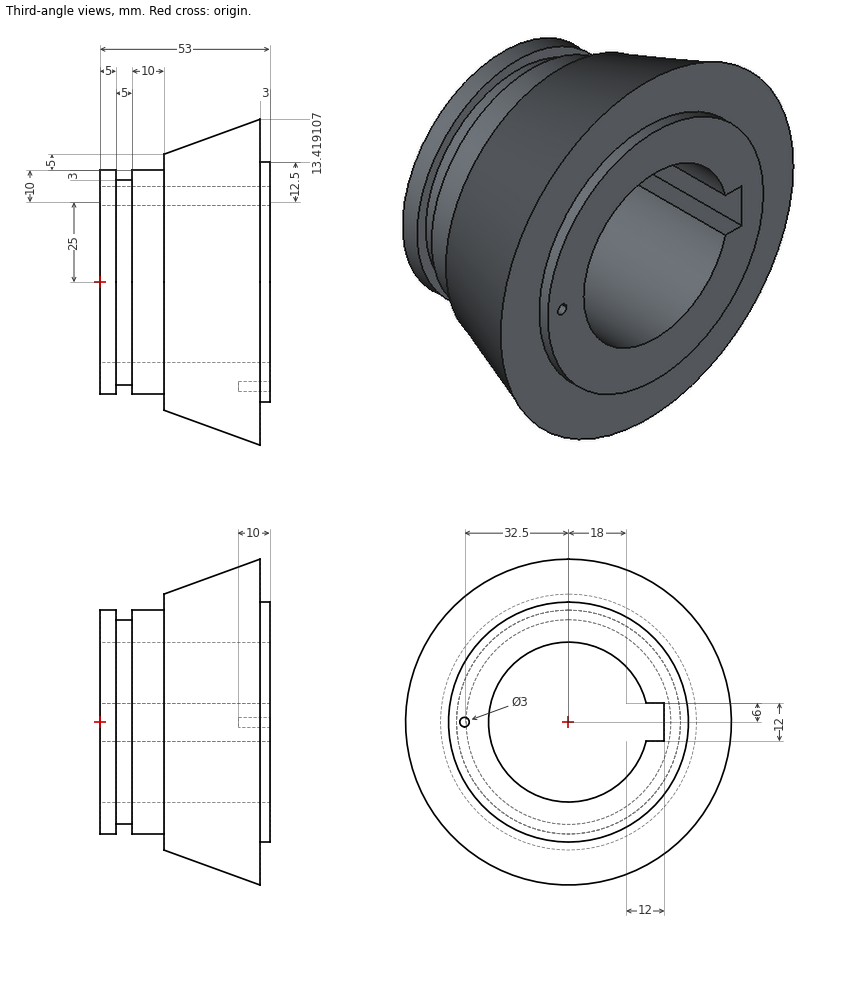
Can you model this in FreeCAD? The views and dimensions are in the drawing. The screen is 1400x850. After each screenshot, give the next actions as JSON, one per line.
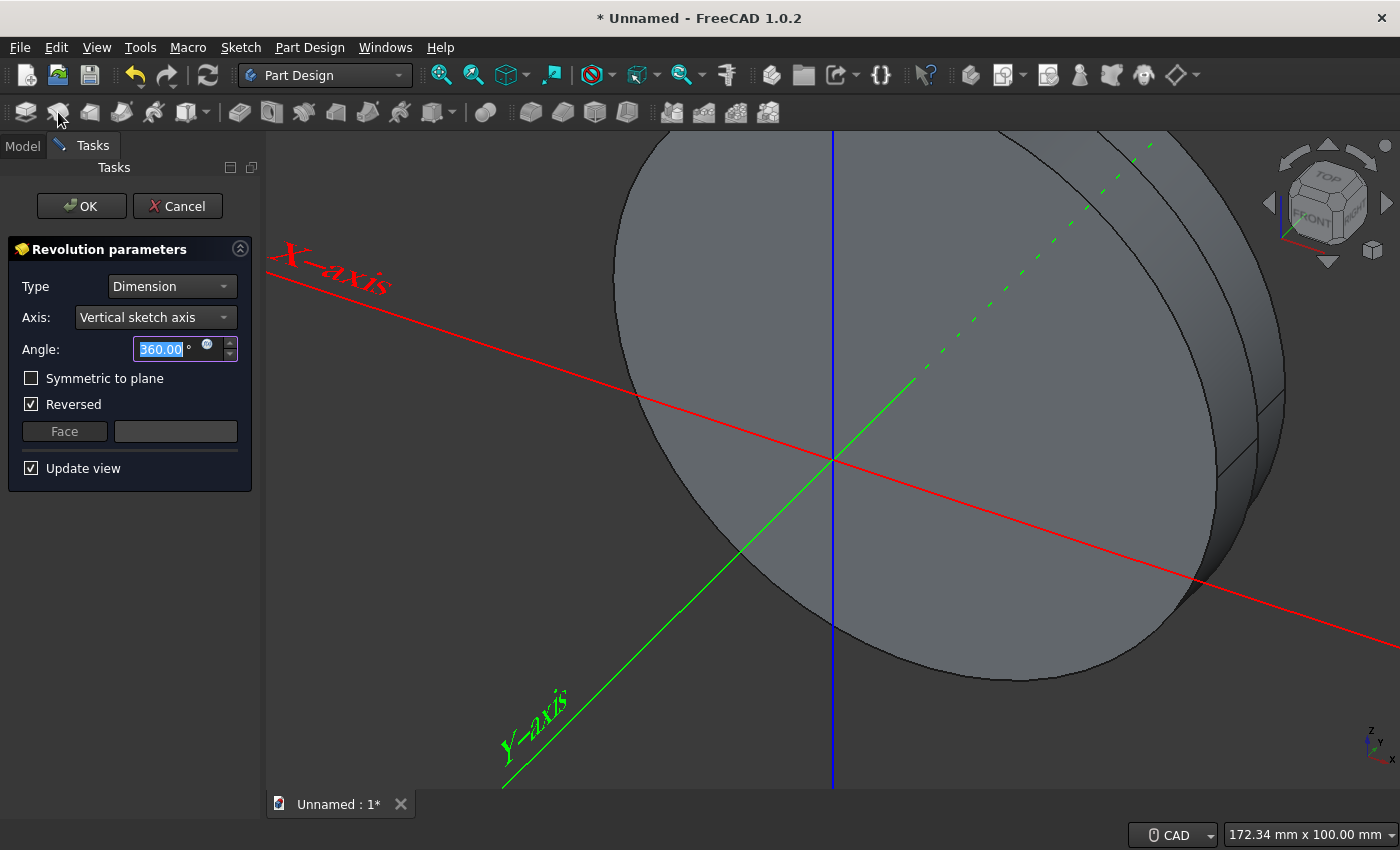
{"action": "left_click", "coordinate": [156, 318]}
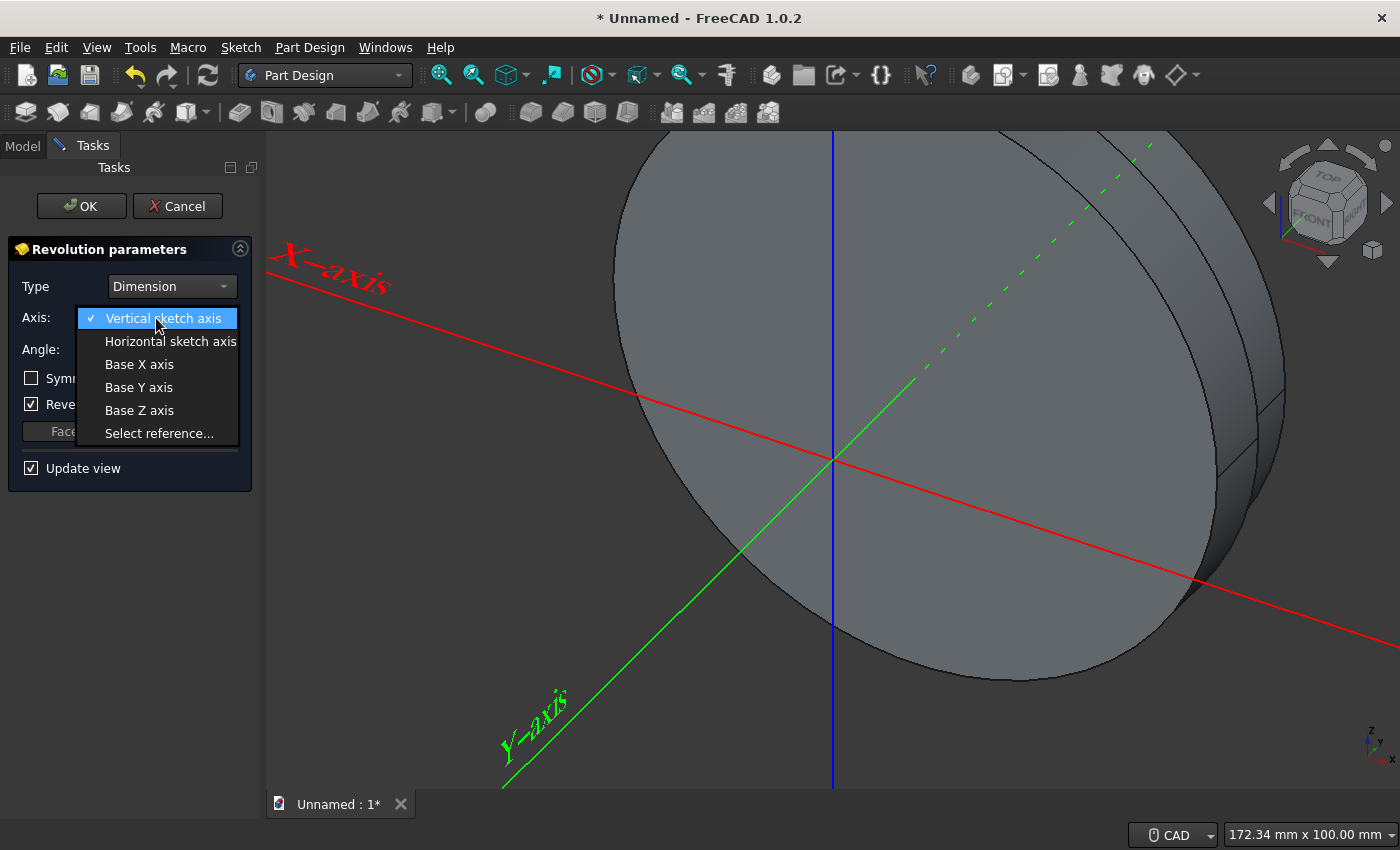
{"action": "left_click", "coordinate": [156, 342]}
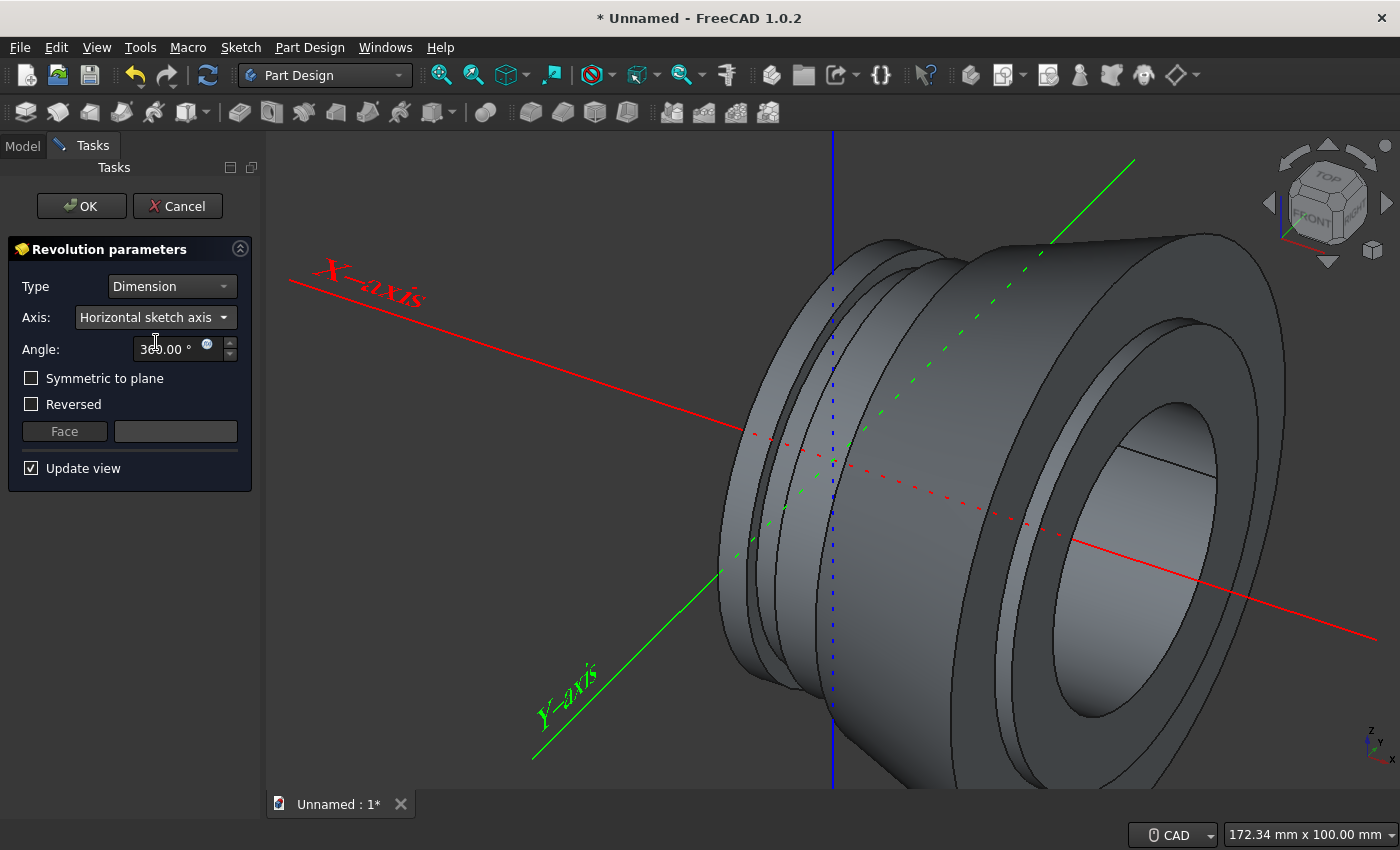
{"action": "left_click", "coordinate": [82, 206]}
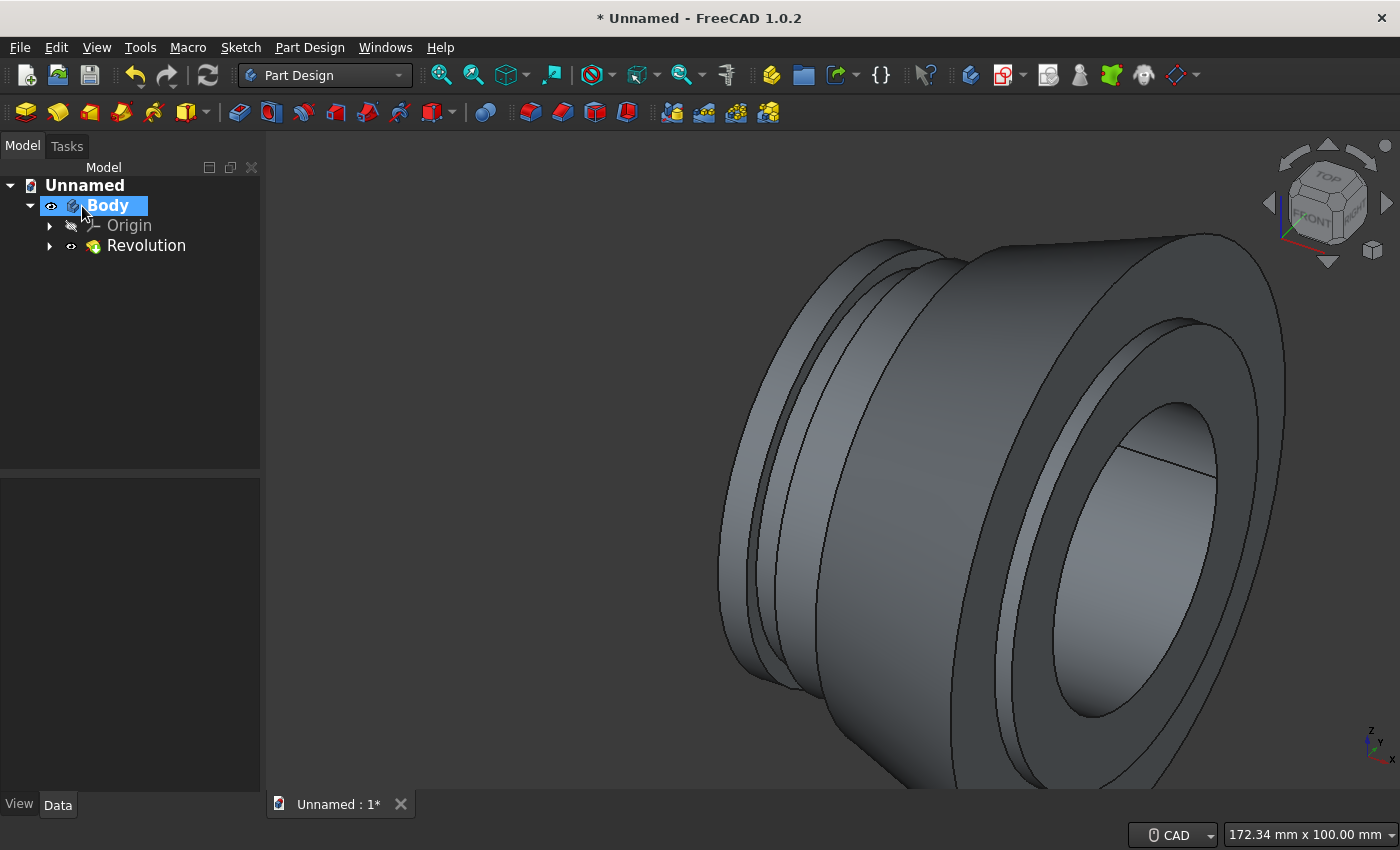
{"action": "left_click", "coordinate": [442, 76]}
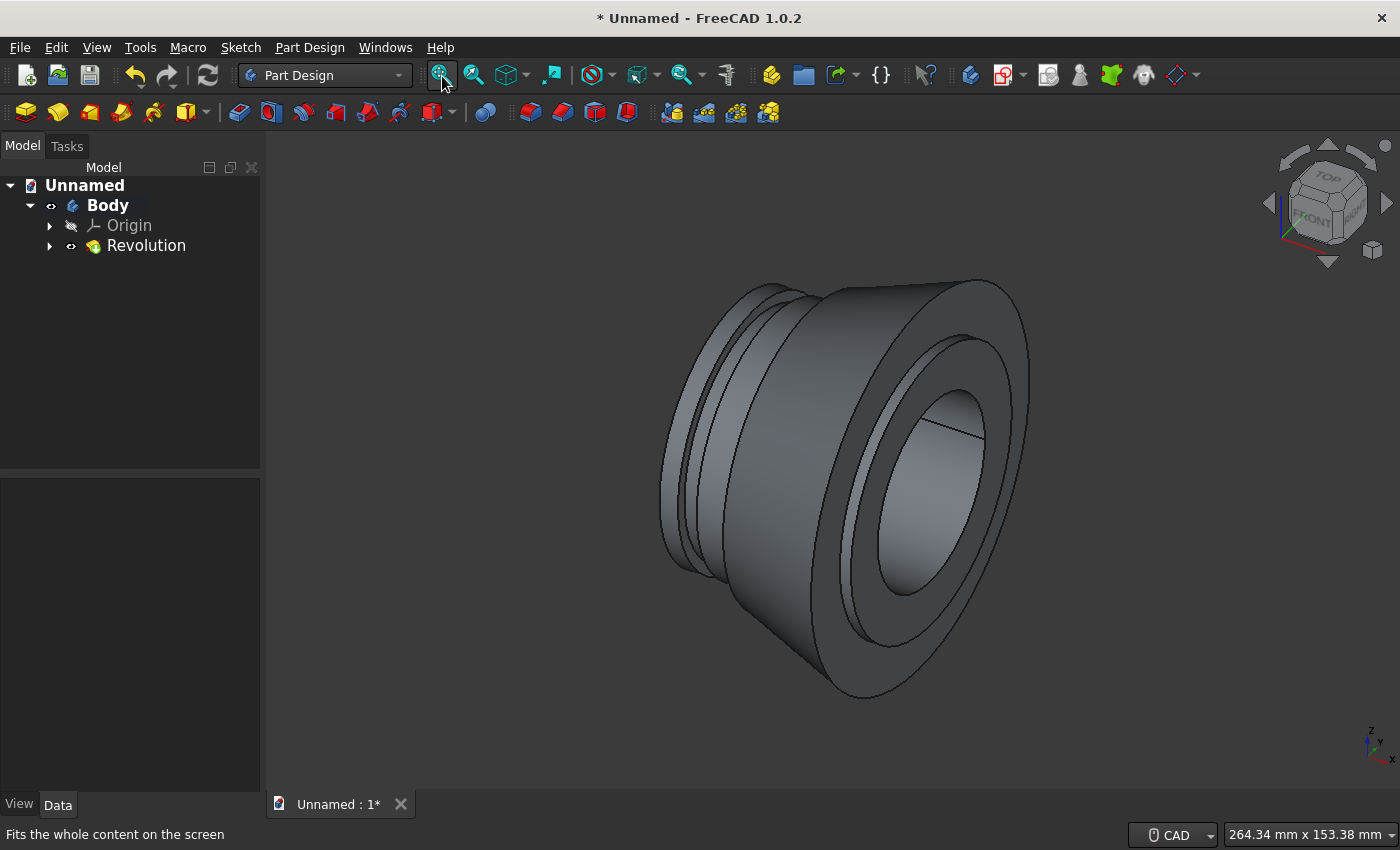
{"action": "left_click", "coordinate": [931, 379]}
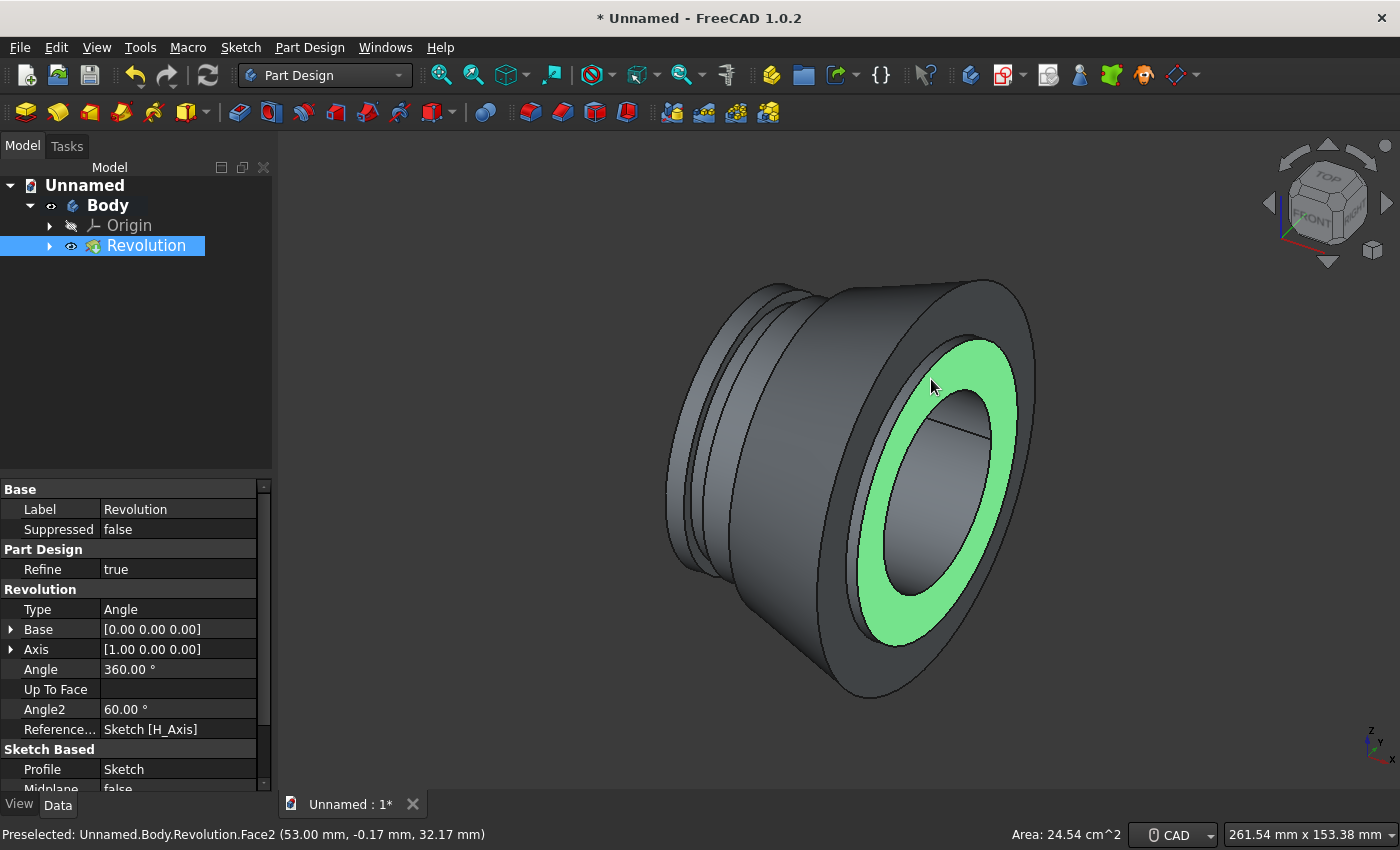
{"action": "left_click", "coordinate": [1004, 76]}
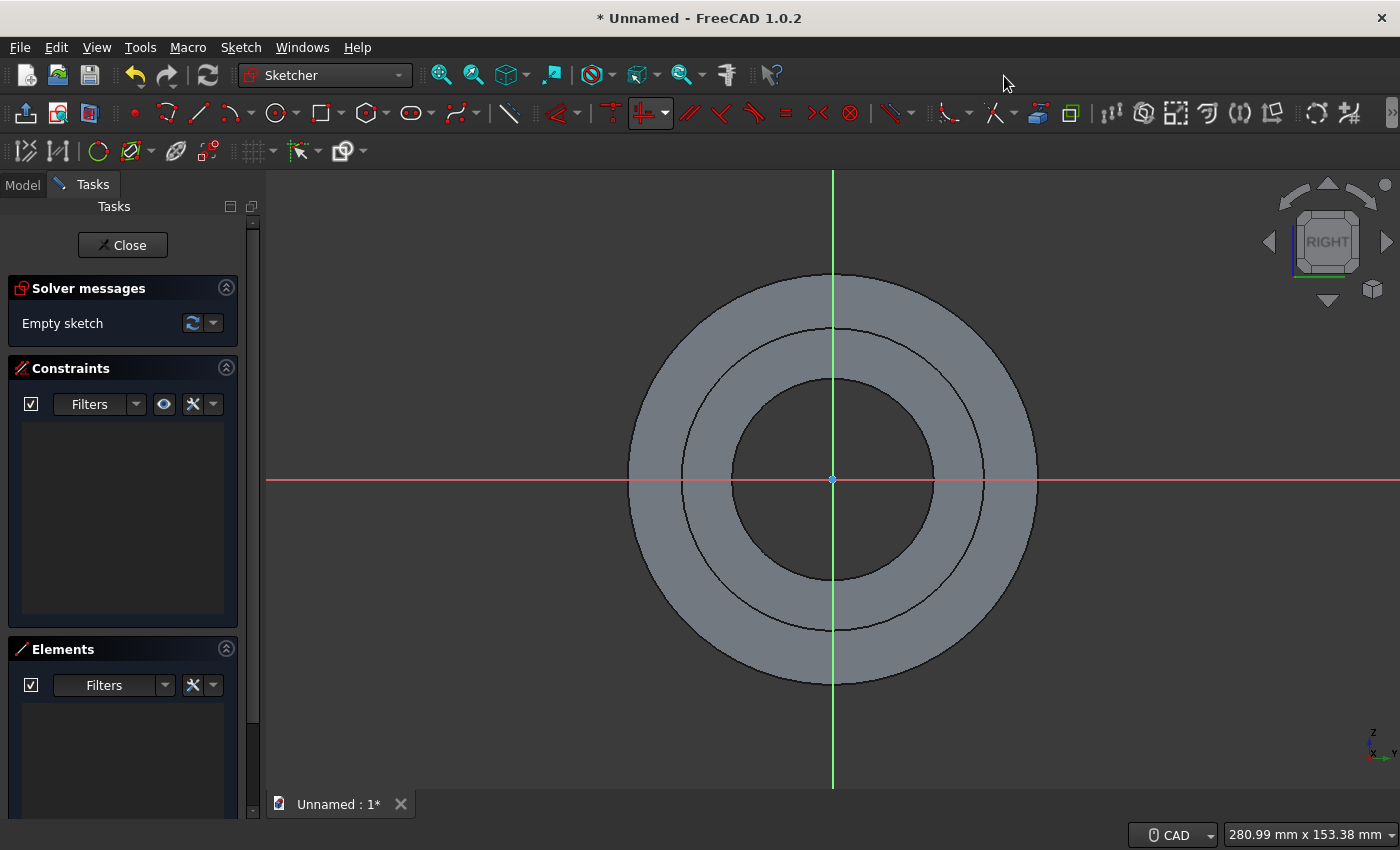
{"action": "scroll", "coordinate": [950, 479], "scroll_direction": "up", "scroll_amount": 11}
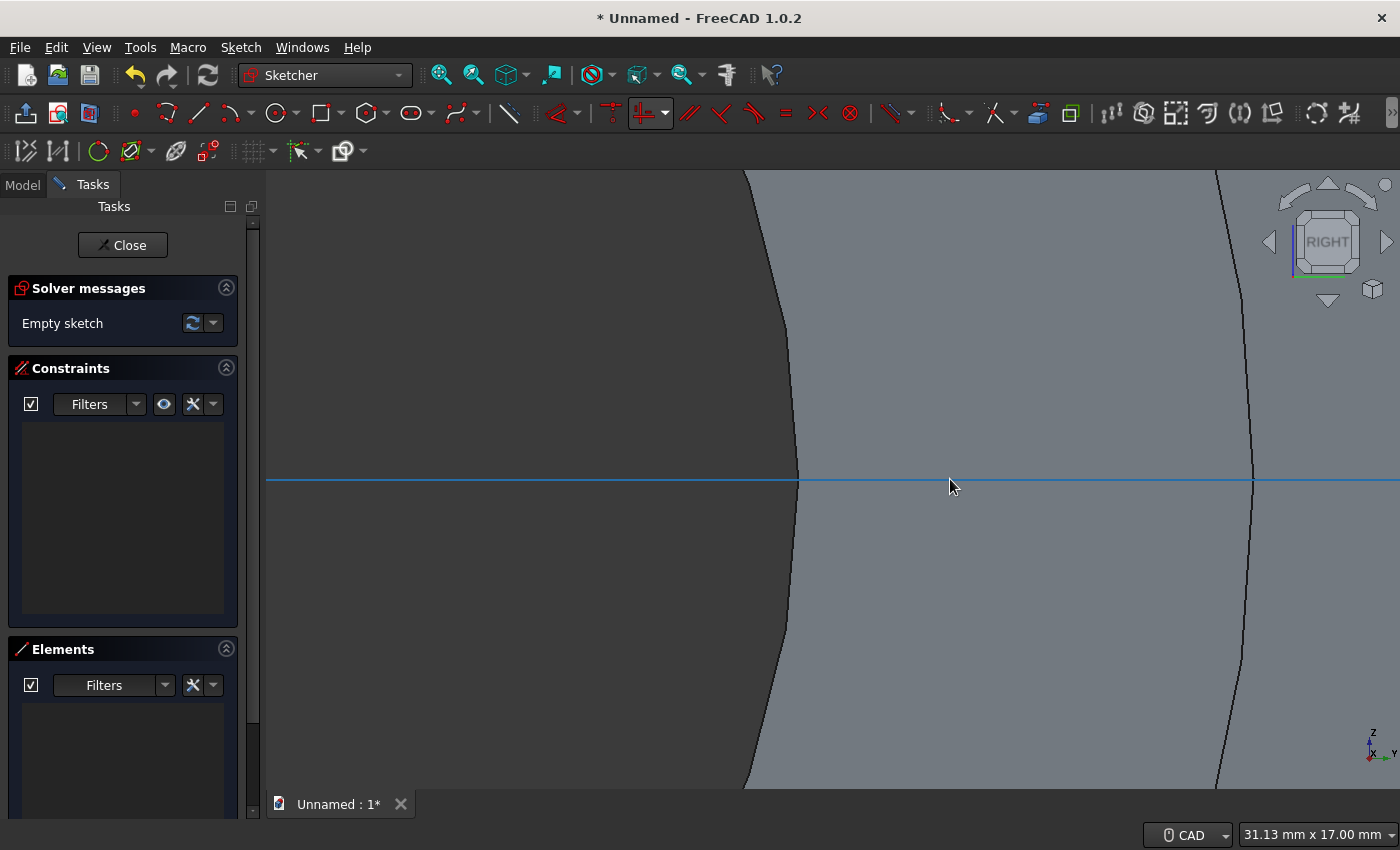
{"action": "left_click", "coordinate": [322, 114]}